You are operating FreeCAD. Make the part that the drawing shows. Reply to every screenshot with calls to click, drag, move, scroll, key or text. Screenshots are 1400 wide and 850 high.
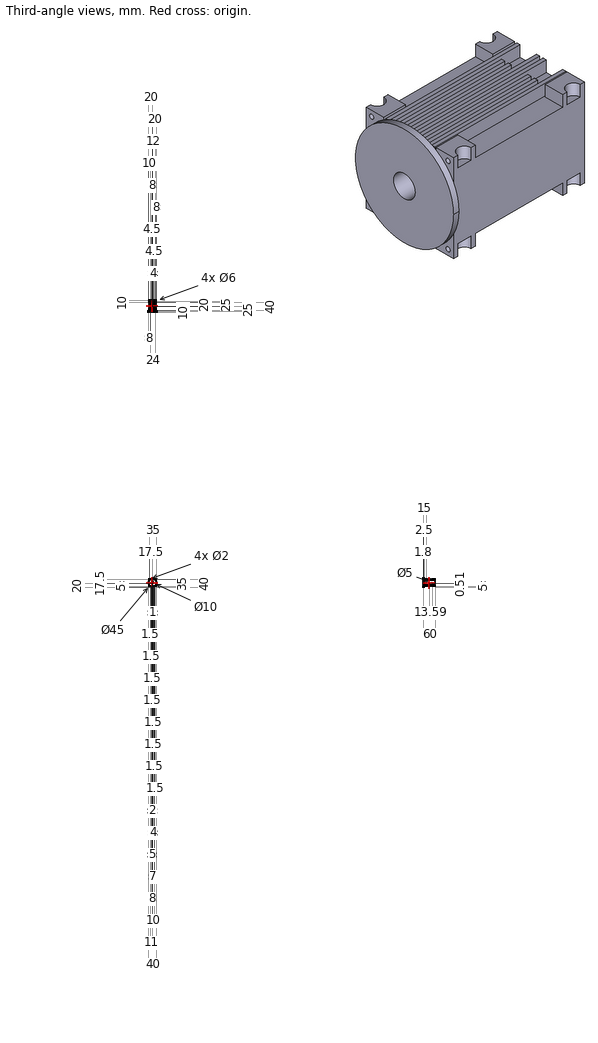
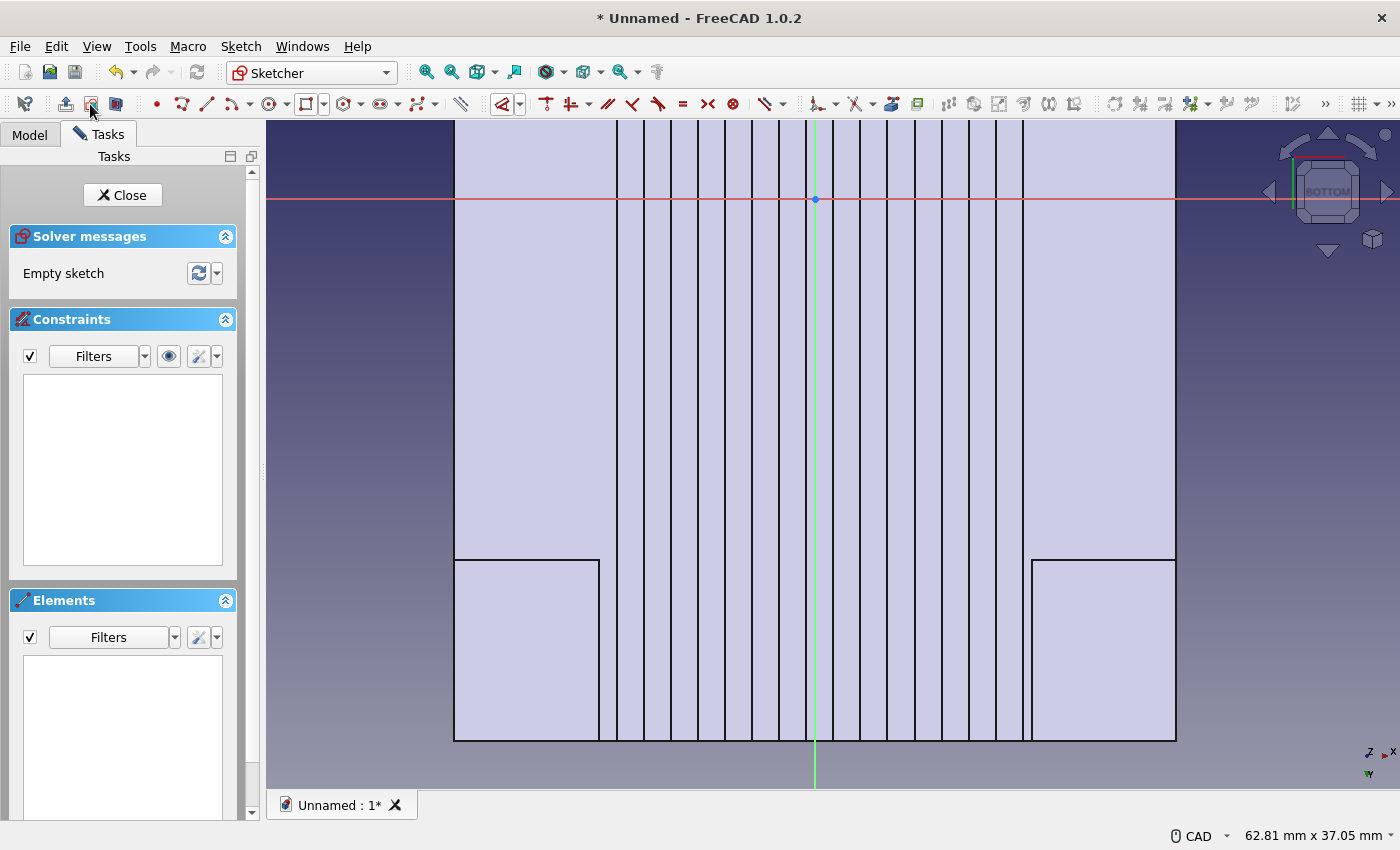
scroll(515, 384, down, 1)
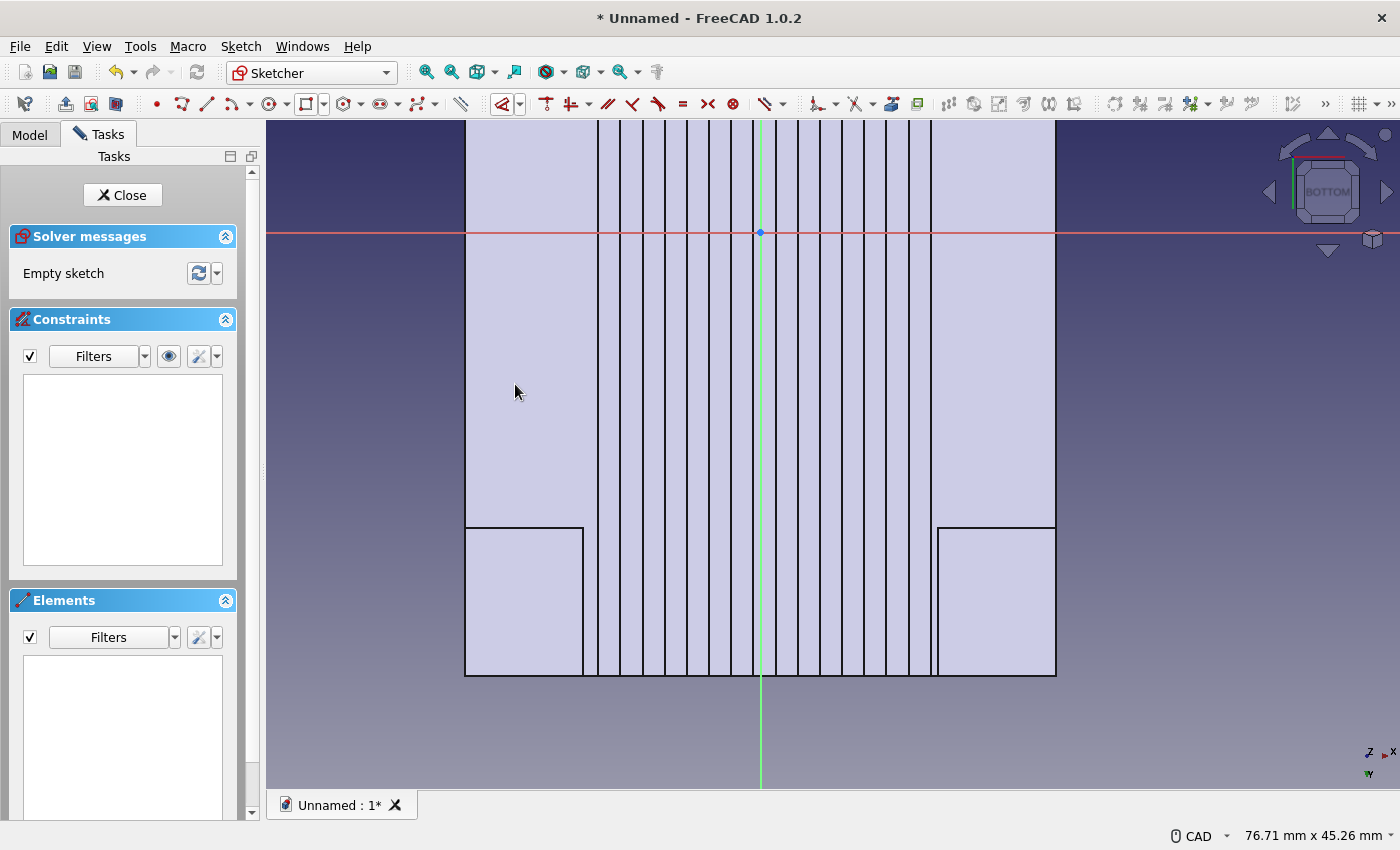
click(306, 104)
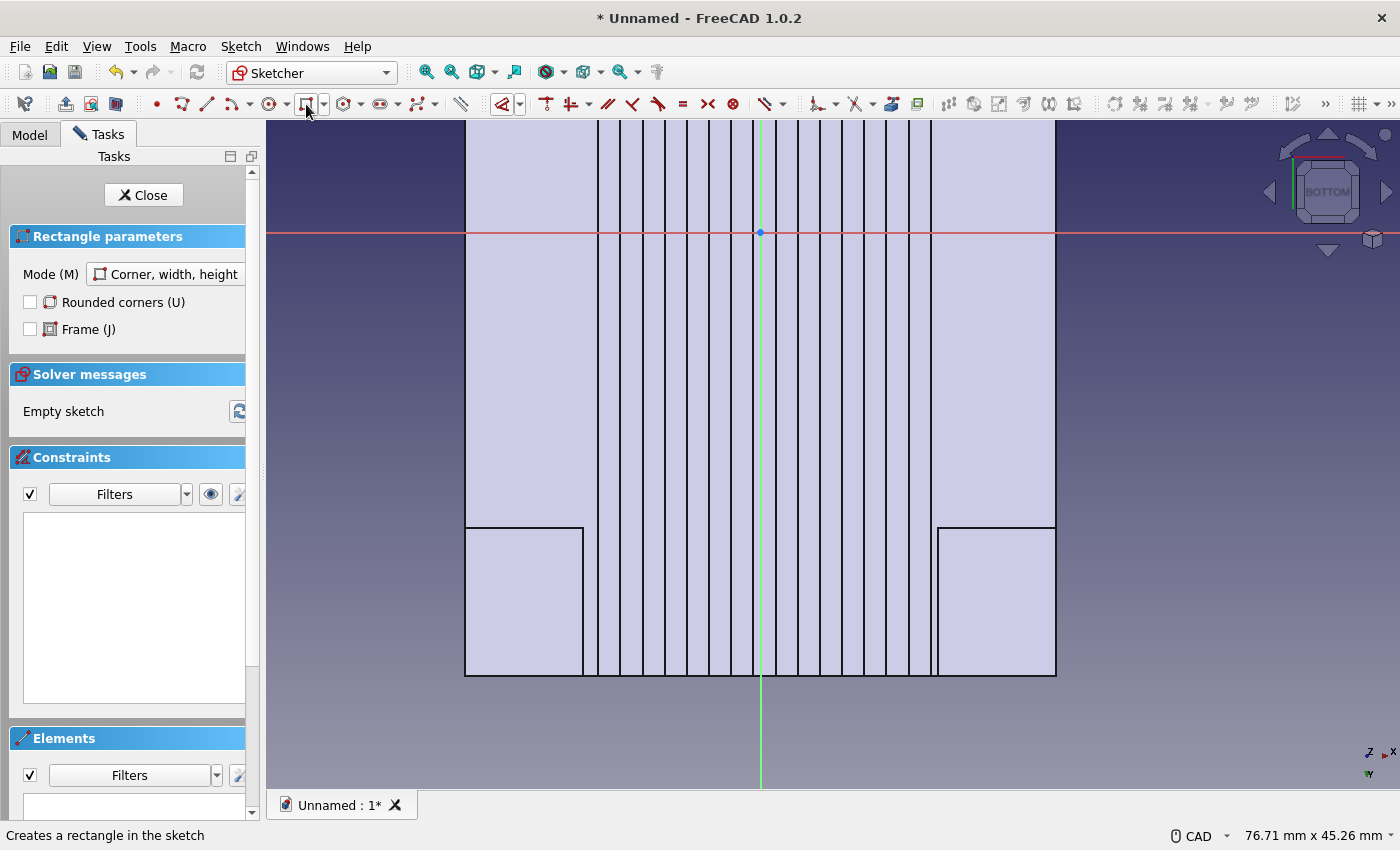
click(820, 528)
click(886, 676)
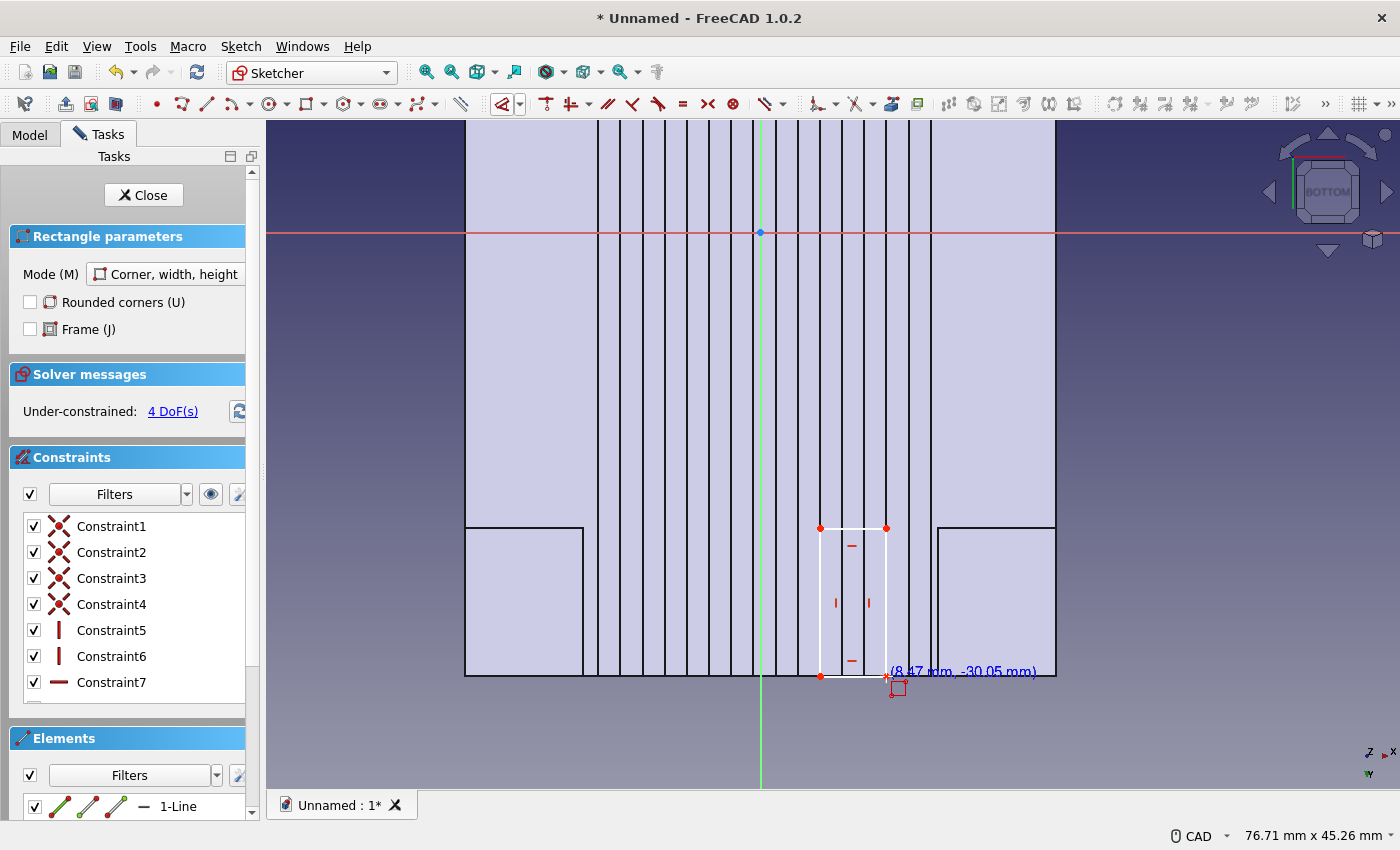
click(643, 528)
click(709, 676)
key(Escape)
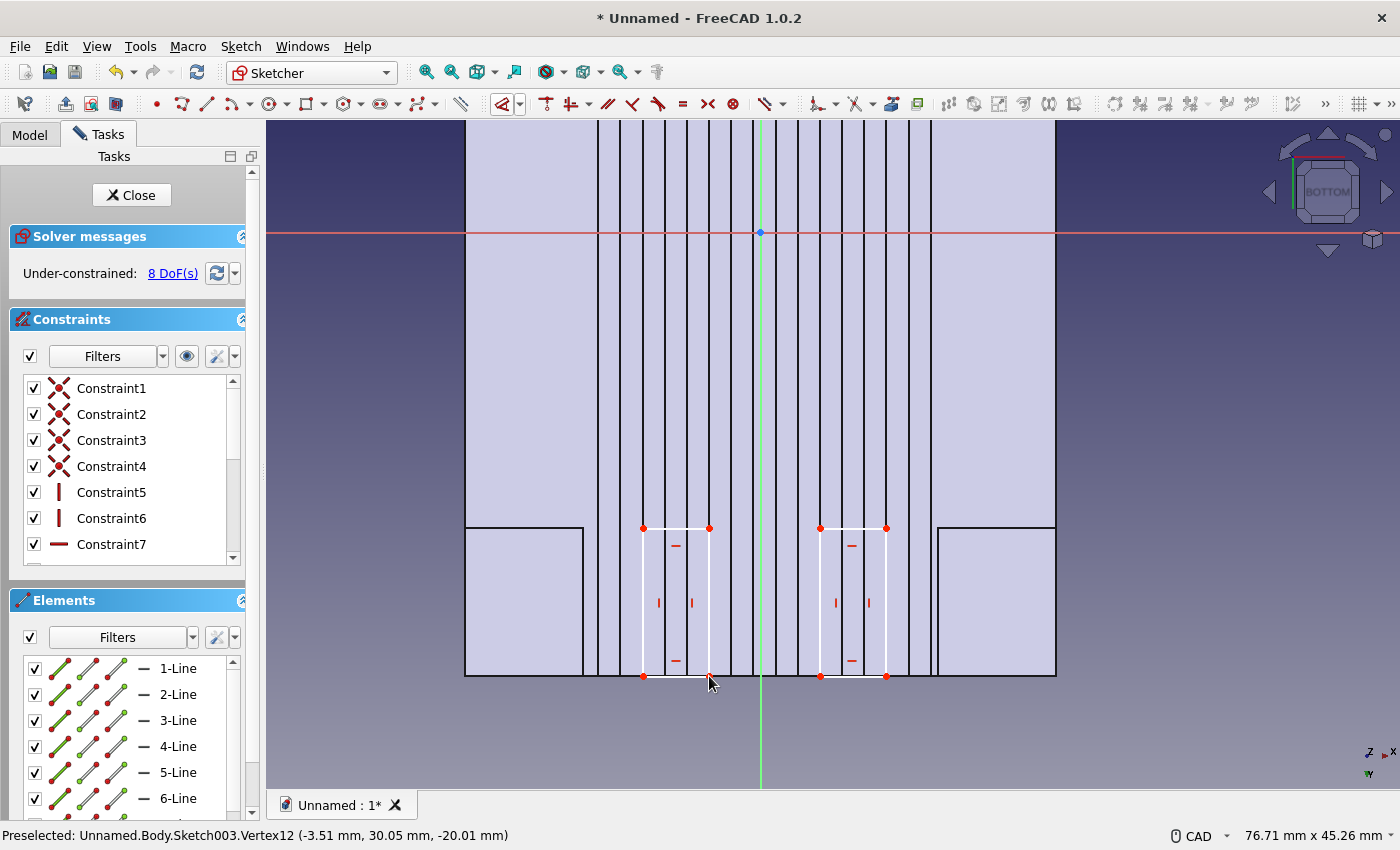
click(820, 573)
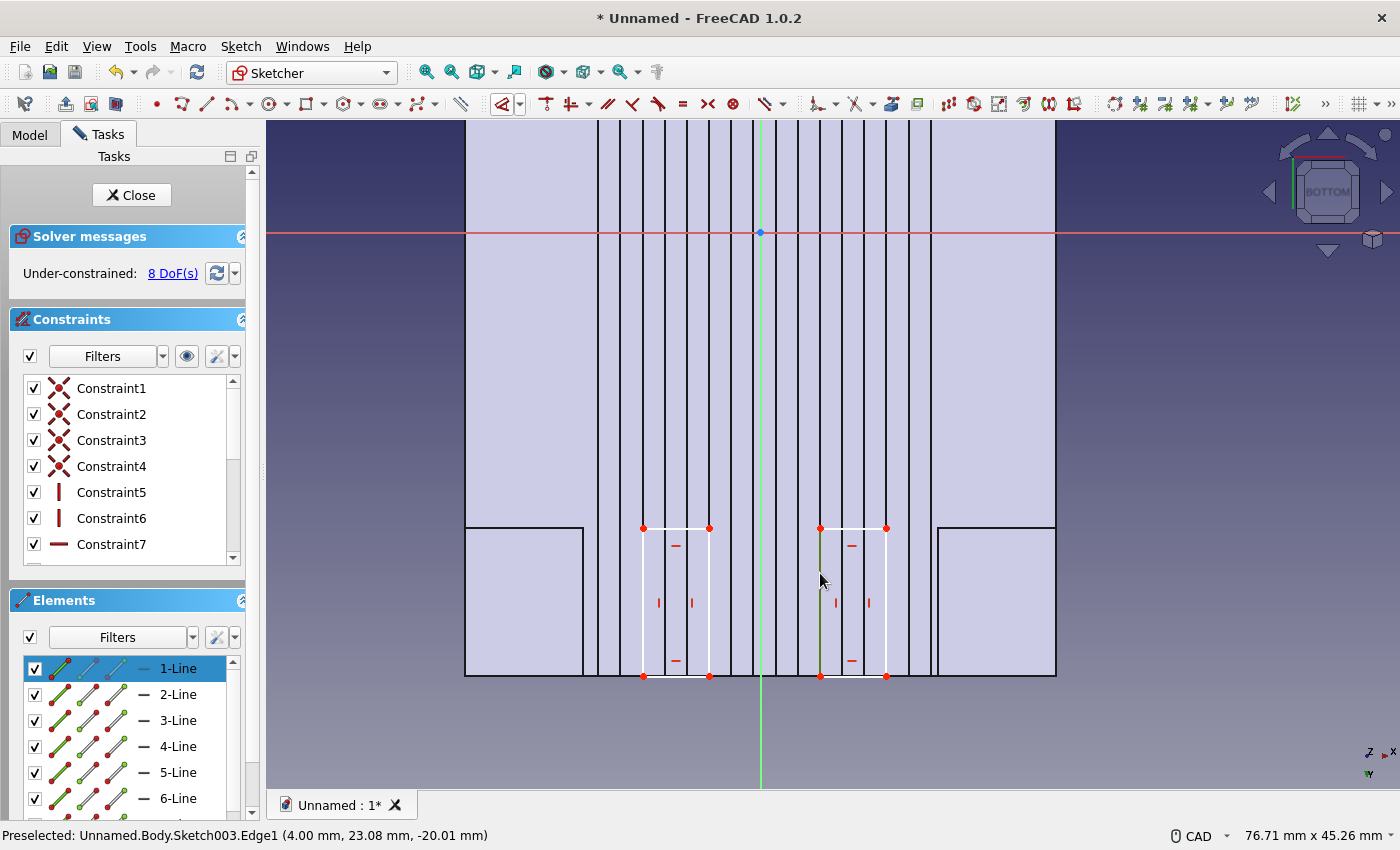
key(i)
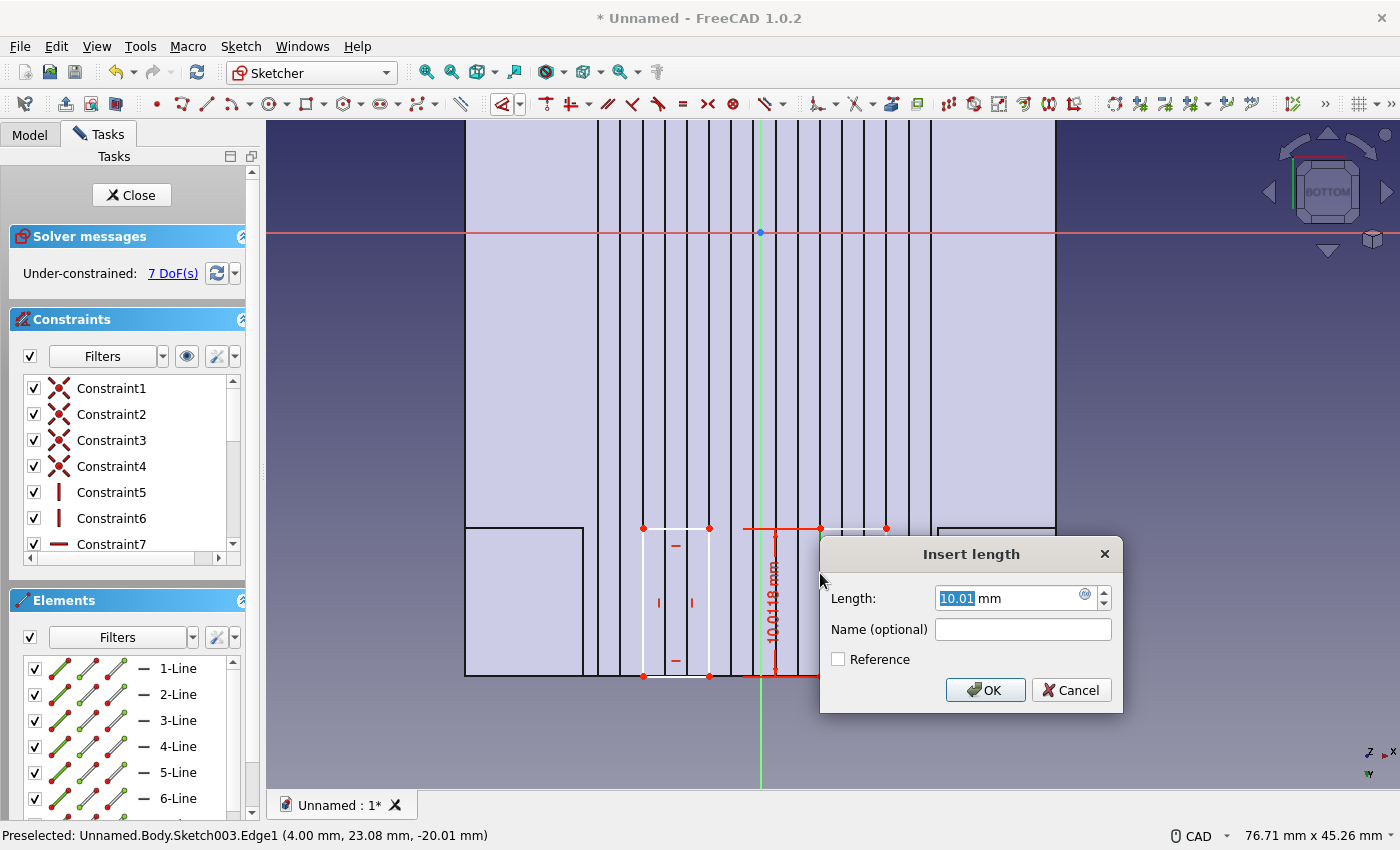
text(10)
key(Return)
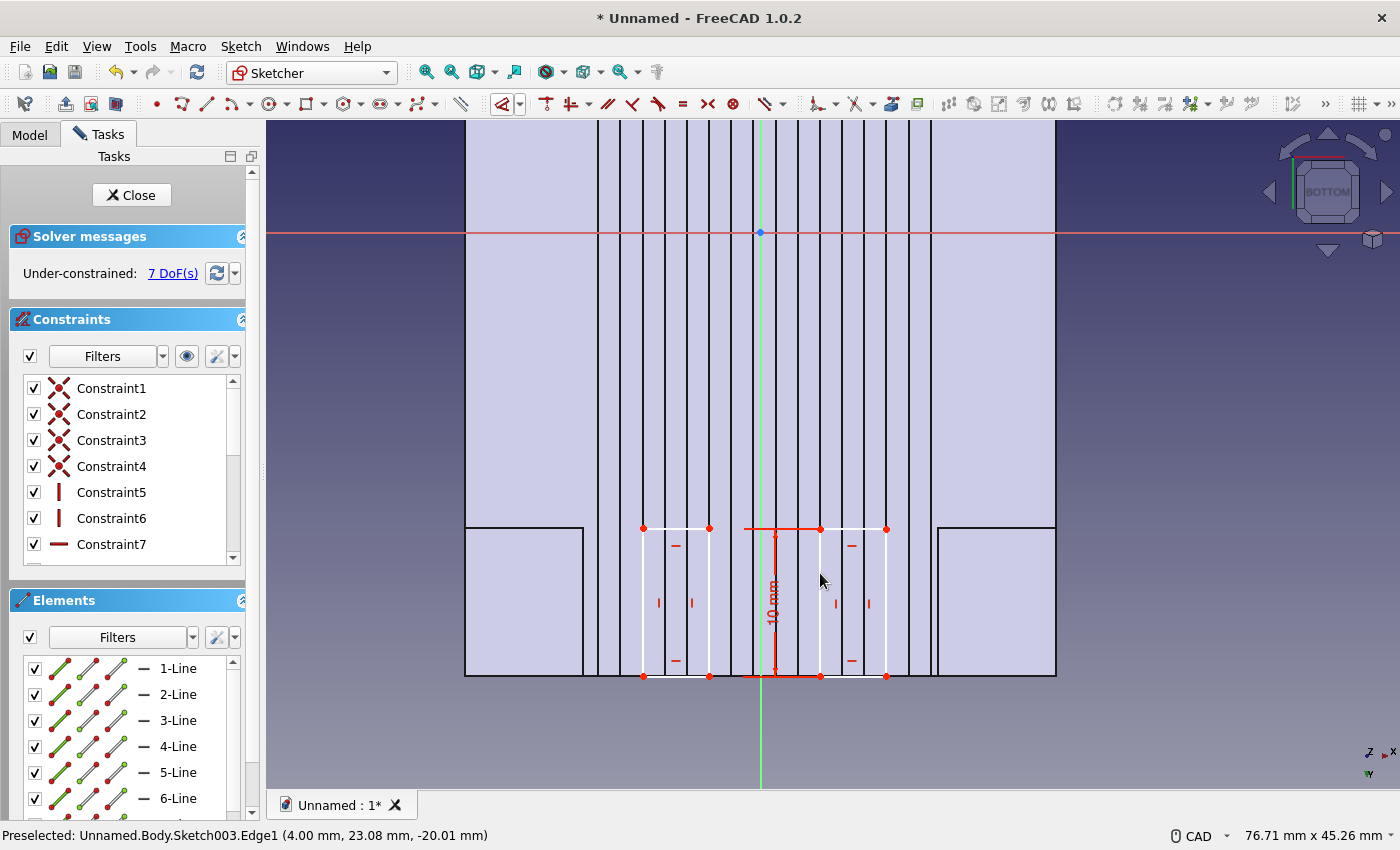
click(643, 573)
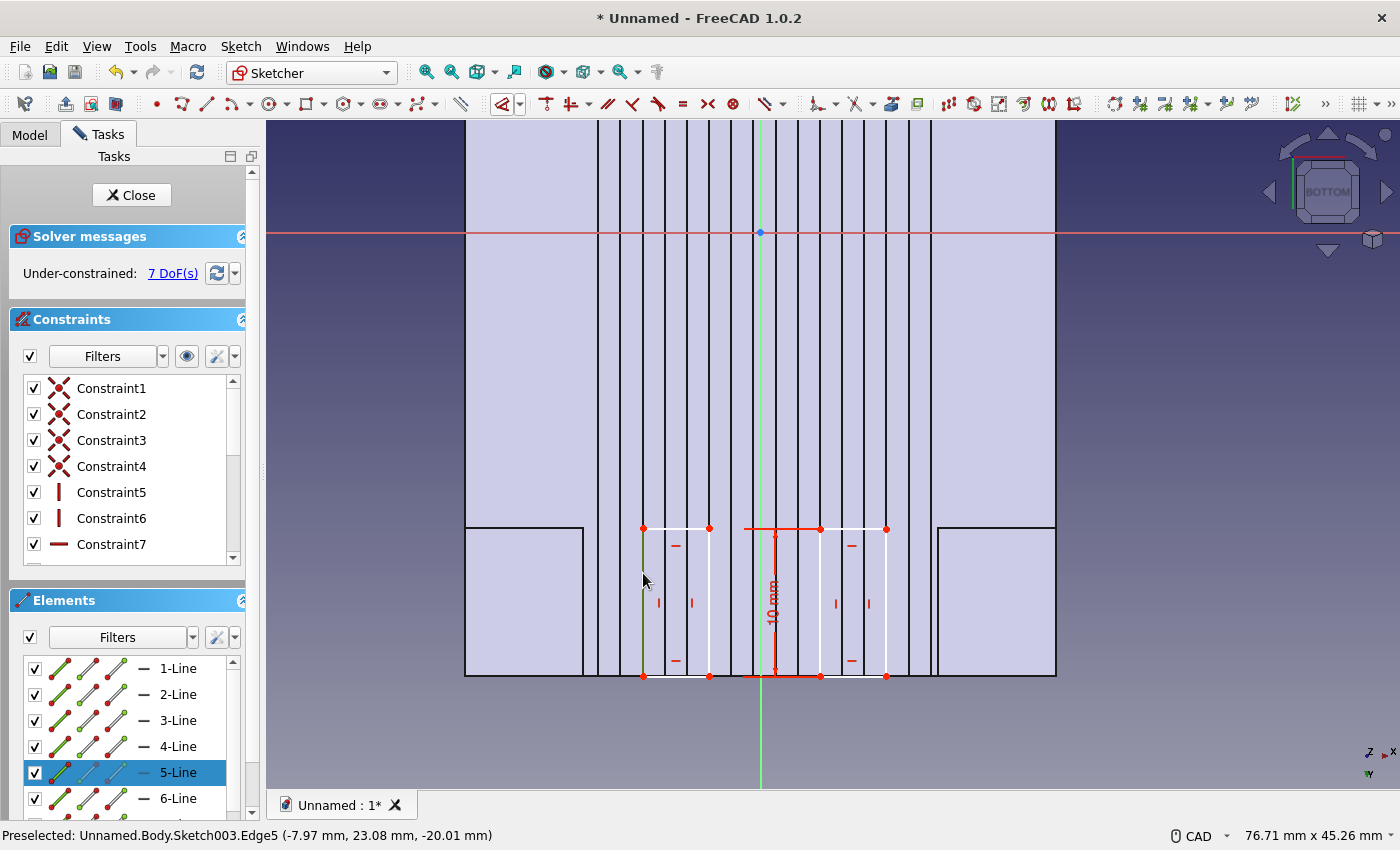
key(i)